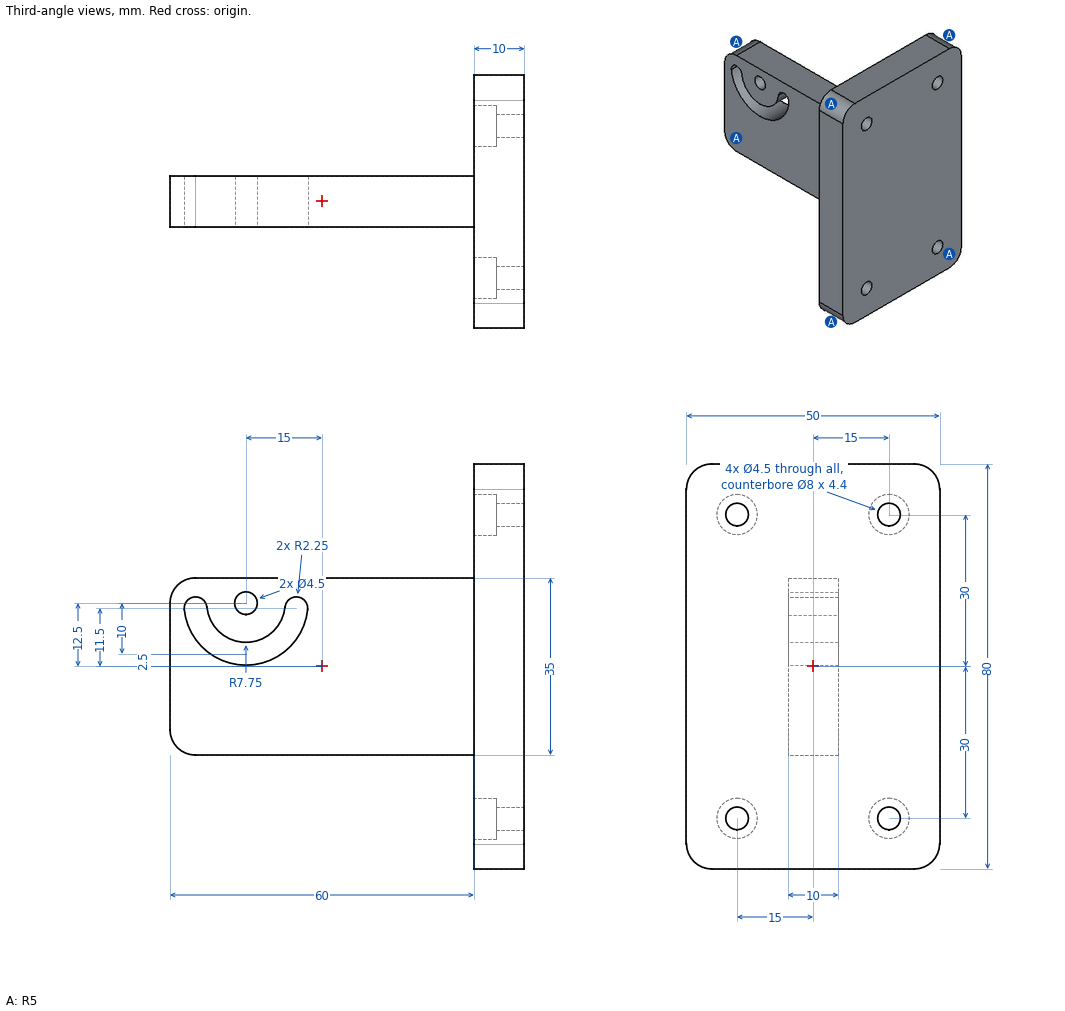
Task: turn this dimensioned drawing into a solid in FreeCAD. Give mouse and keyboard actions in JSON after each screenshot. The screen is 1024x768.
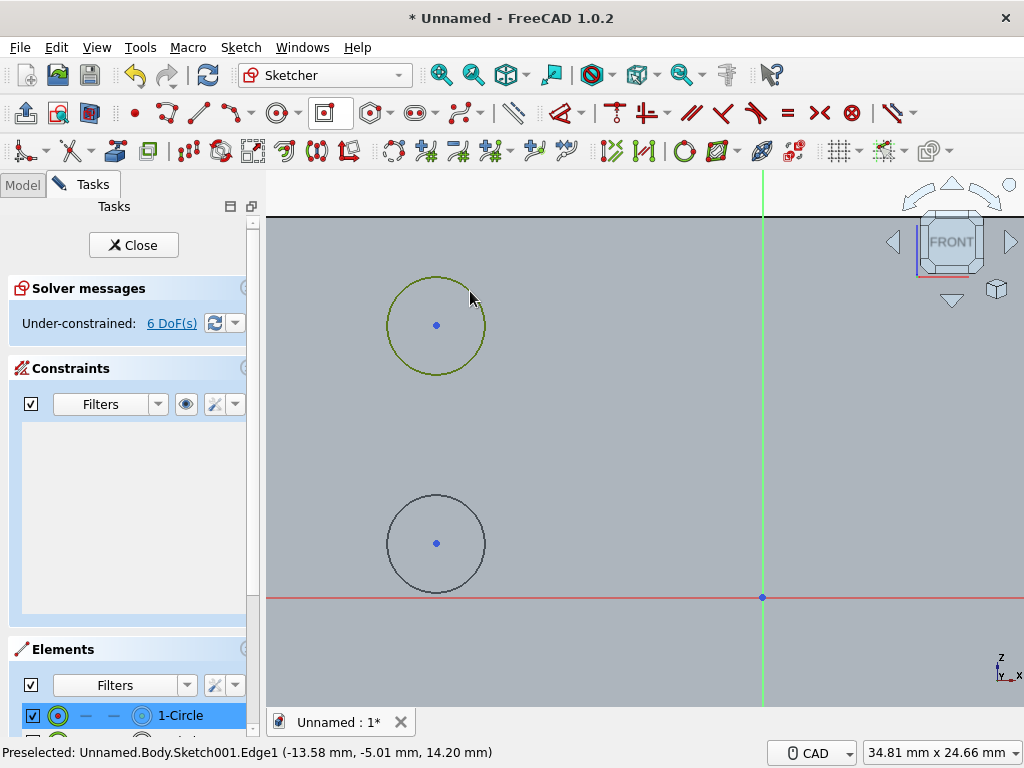
{"action": "left_click", "coordinate": [470, 509]}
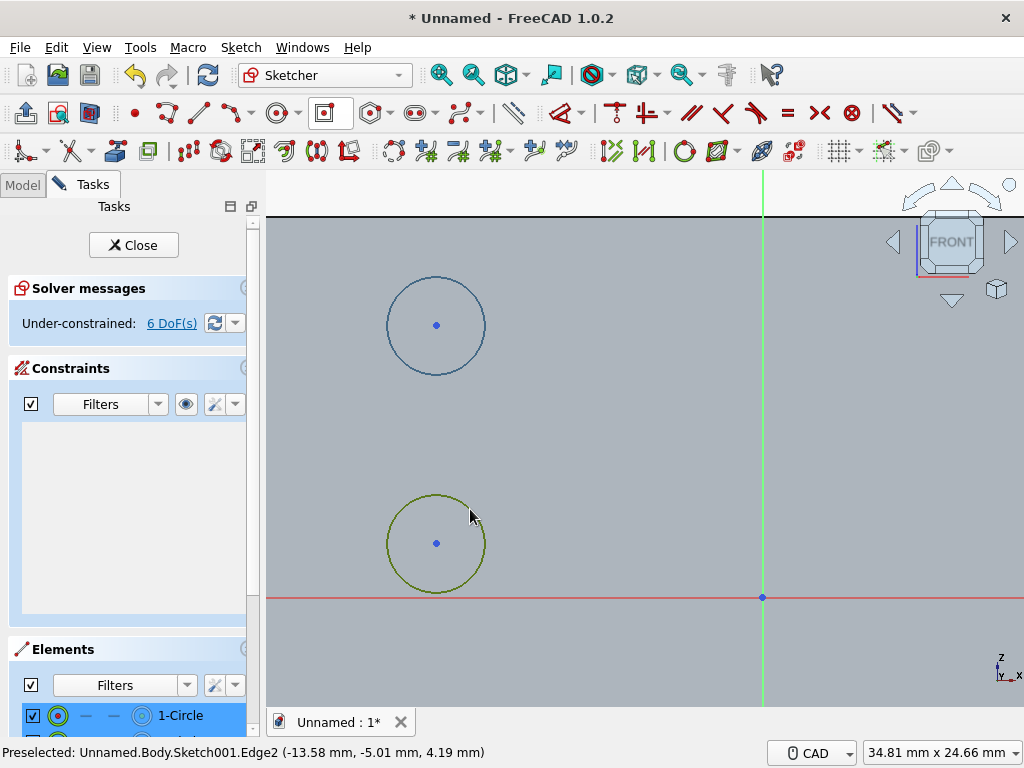
{"action": "left_click", "coordinate": [788, 114]}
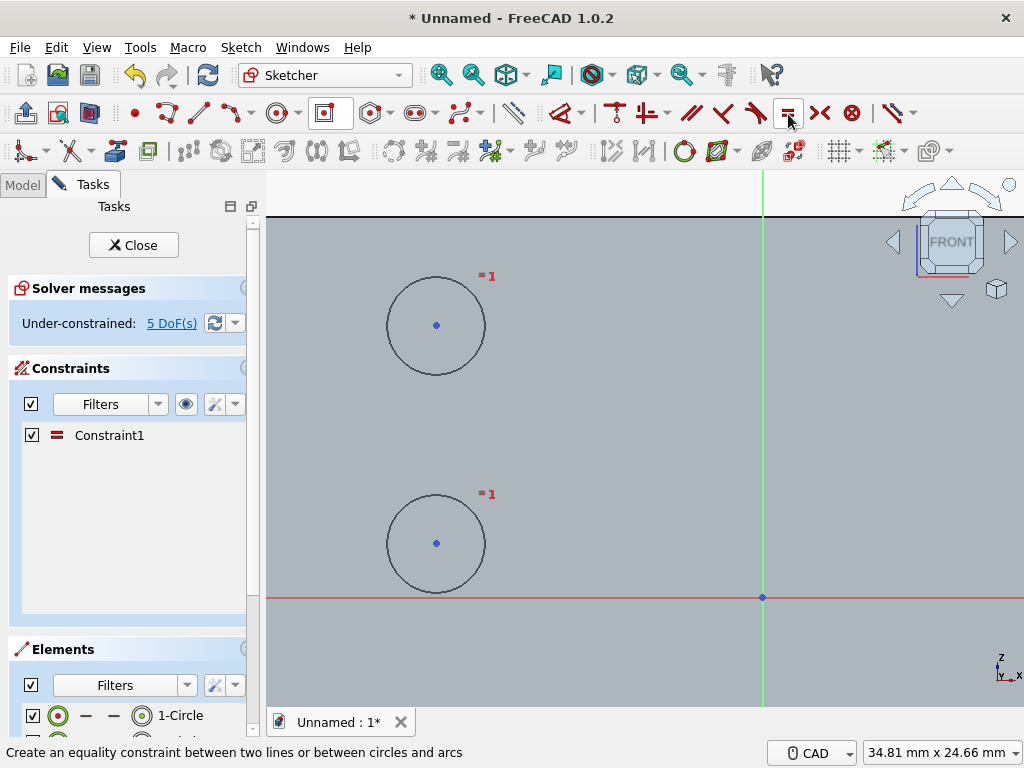
{"action": "left_click", "coordinate": [436, 326]}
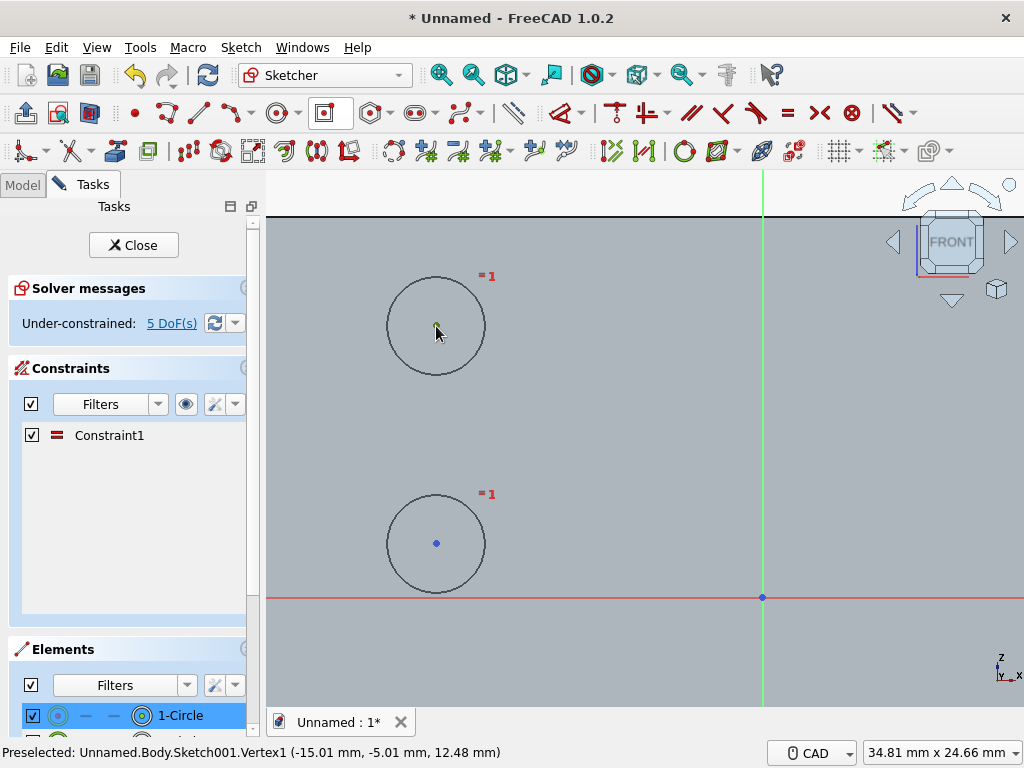
{"action": "left_click", "coordinate": [436, 544]}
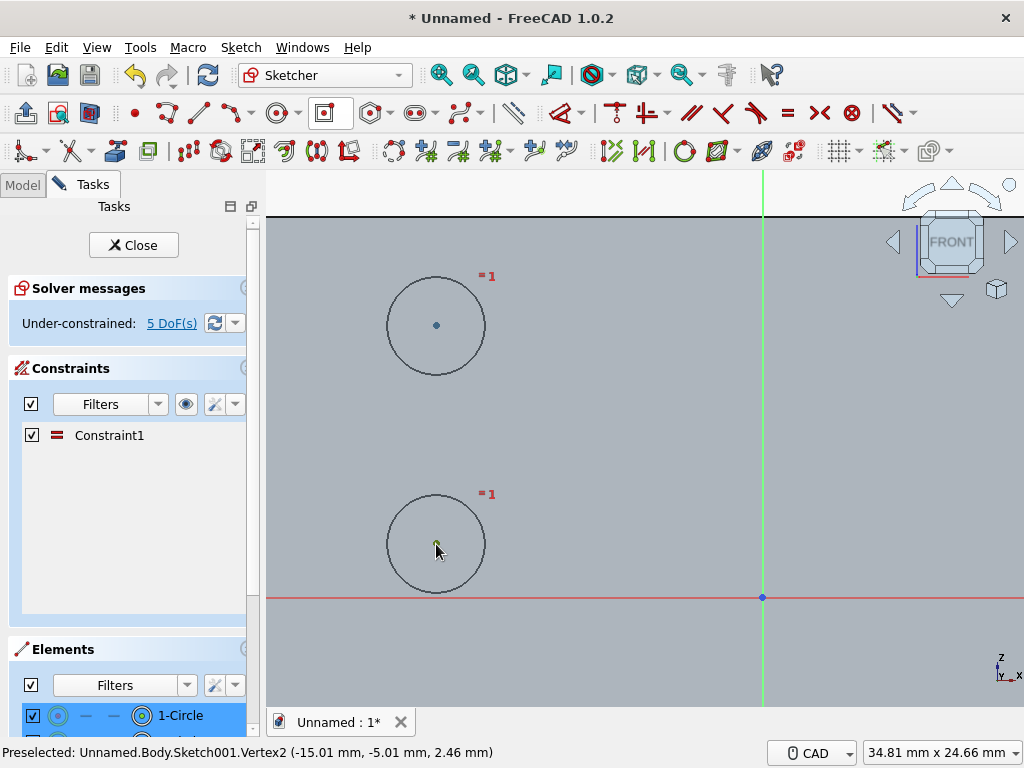
{"action": "left_click", "coordinate": [670, 114]}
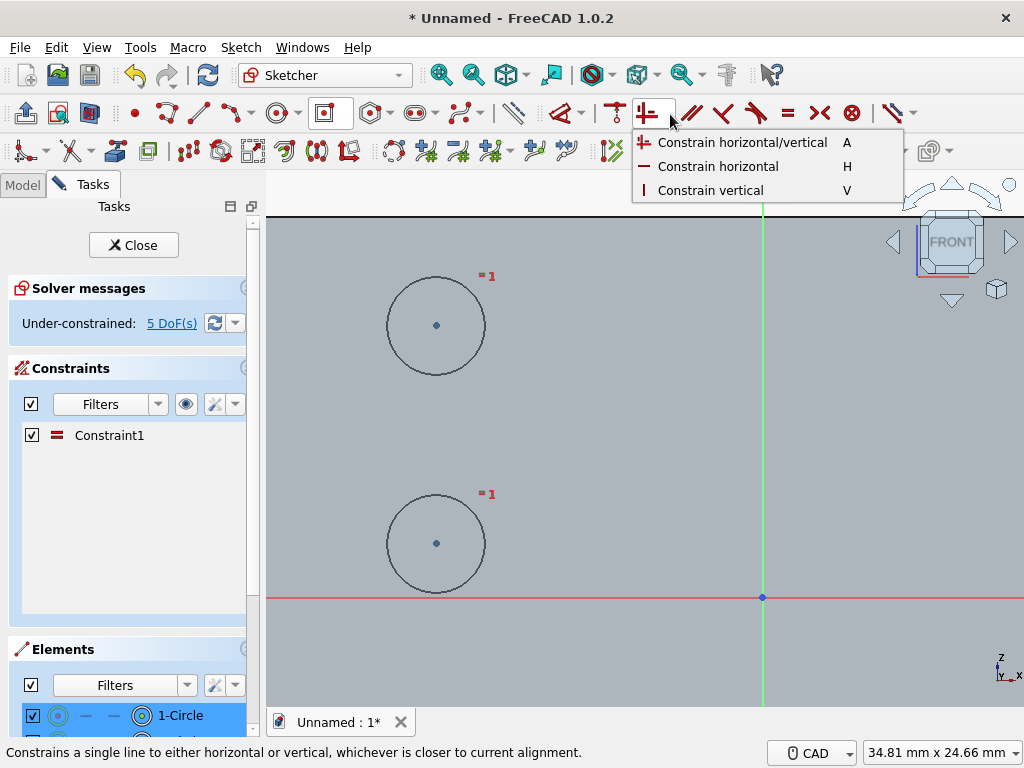
{"action": "left_click", "coordinate": [768, 190]}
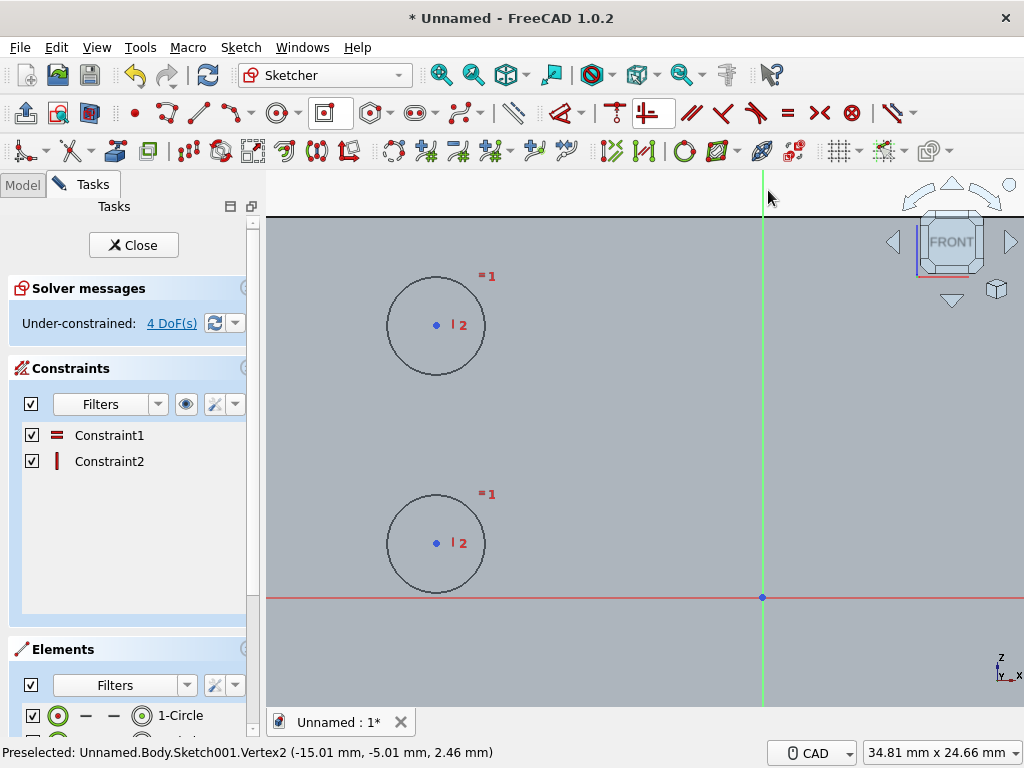
{"action": "left_click", "coordinate": [560, 114]}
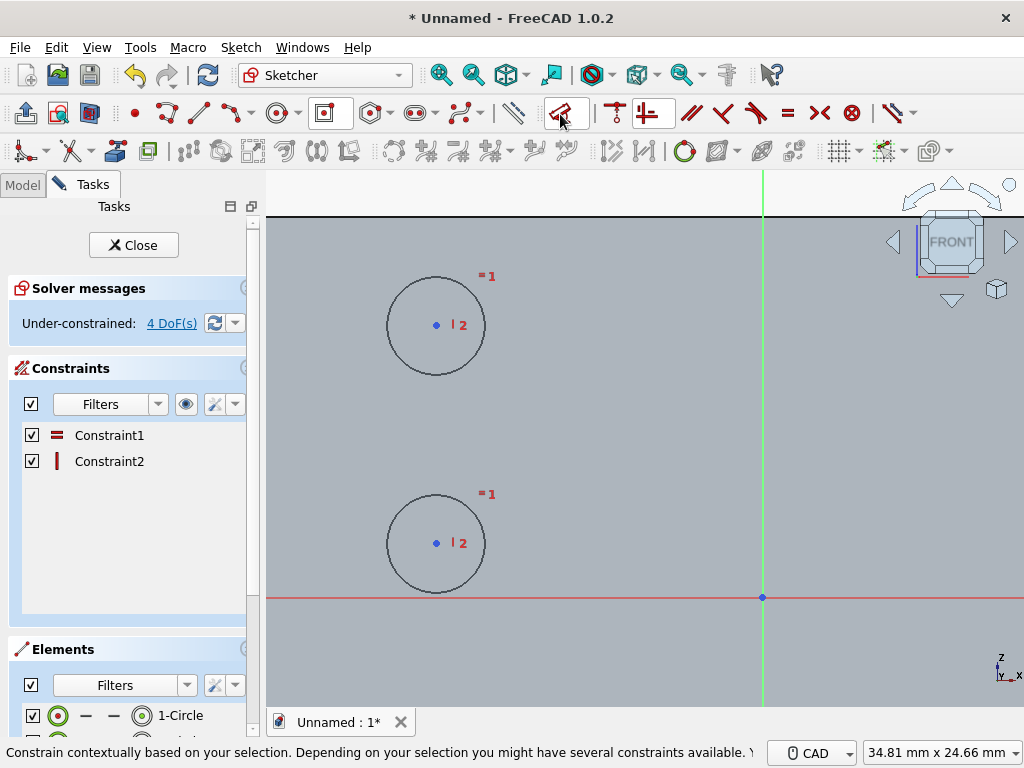
{"action": "left_click", "coordinate": [470, 291]}
{"action": "left_click", "coordinate": [492, 268]}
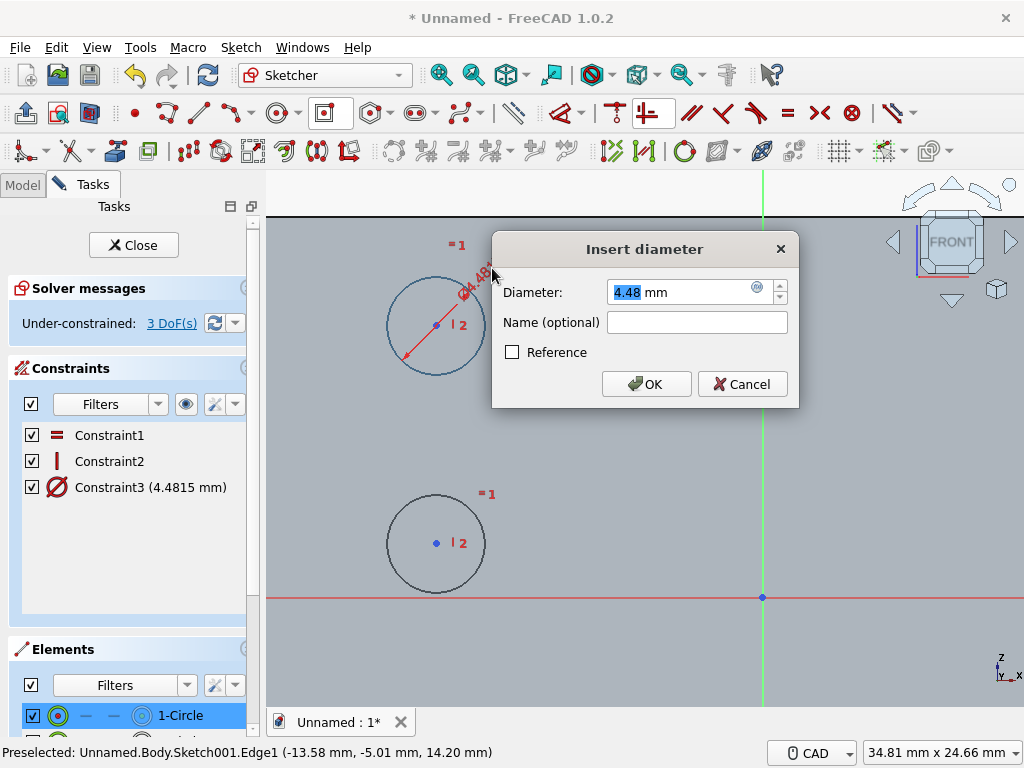
{"action": "type", "text": "4.5"}
{"action": "key", "text": "Return"}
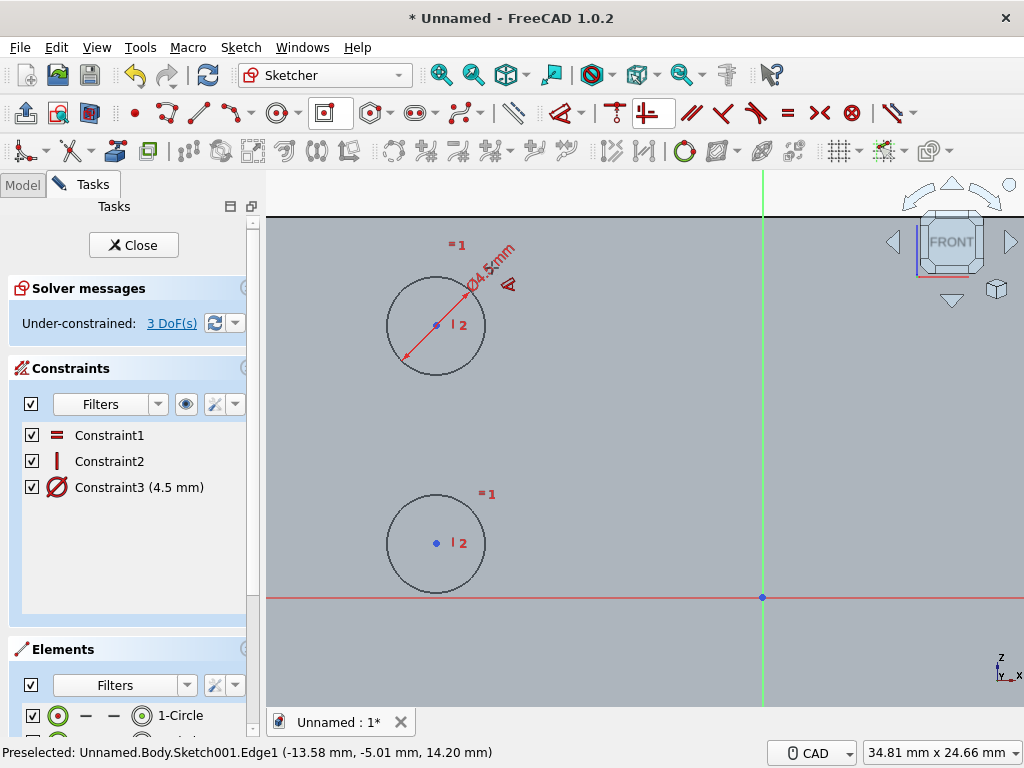
{"action": "left_click", "coordinate": [436, 326]}
{"action": "left_click", "coordinate": [599, 632]}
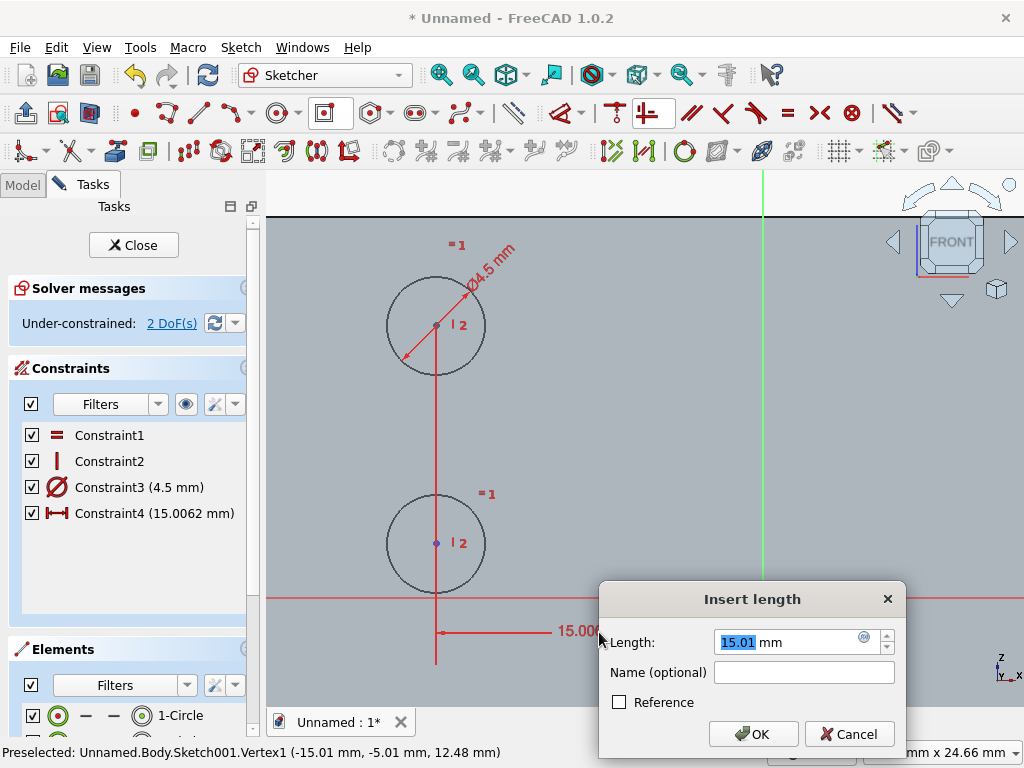
{"action": "type", "text": "15"}
{"action": "key", "text": "Return"}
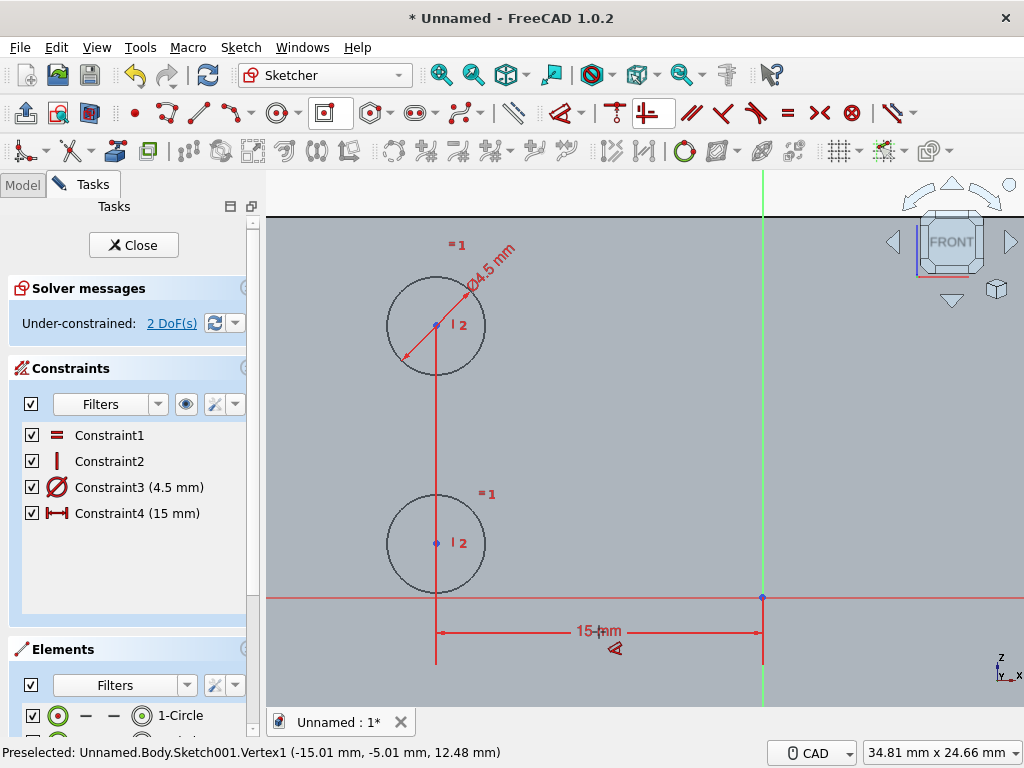
{"action": "left_click", "coordinate": [436, 544]}
{"action": "left_click", "coordinate": [797, 571]}